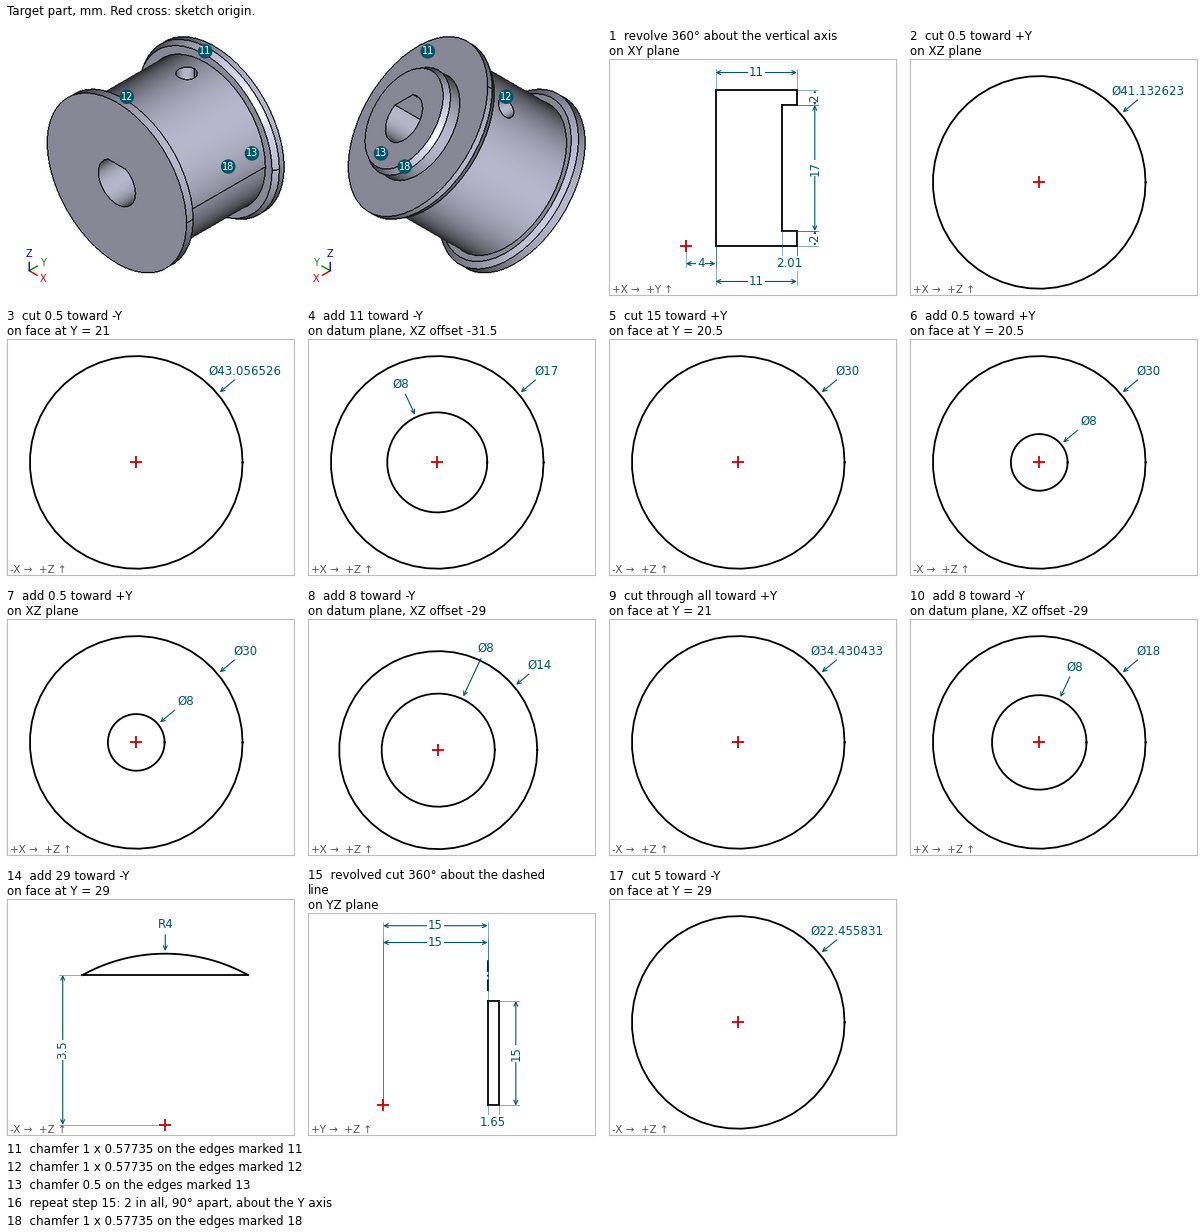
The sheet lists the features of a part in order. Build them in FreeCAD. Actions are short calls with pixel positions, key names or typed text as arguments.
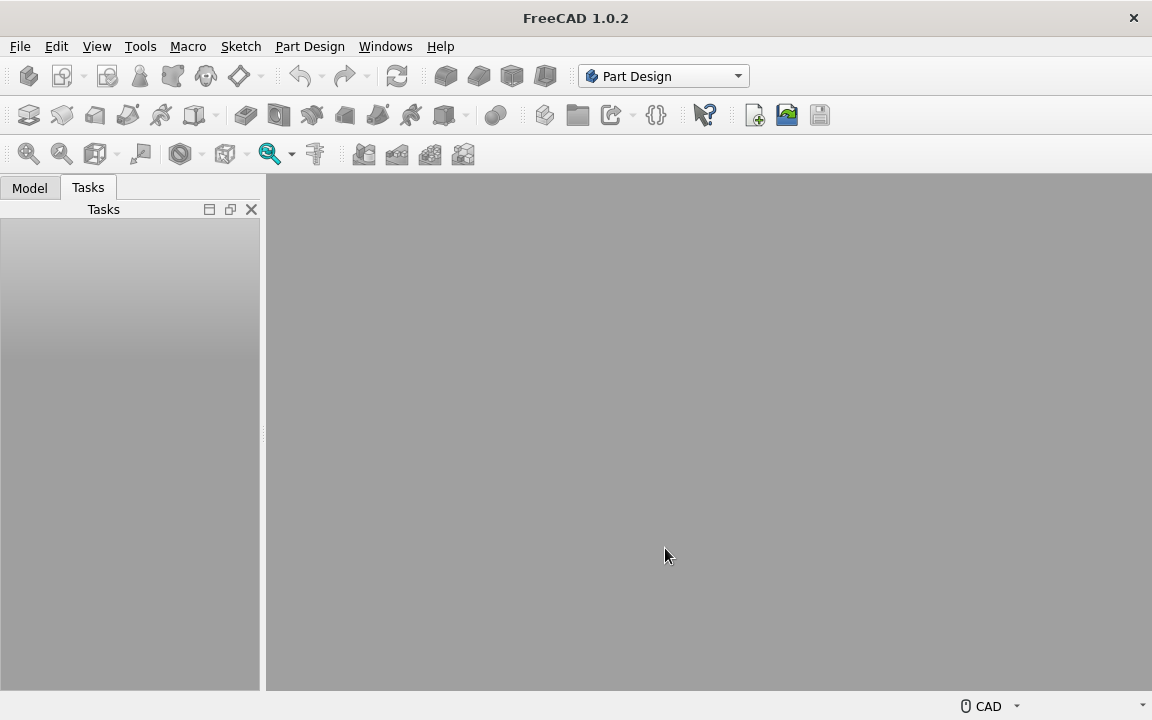
click(754, 116)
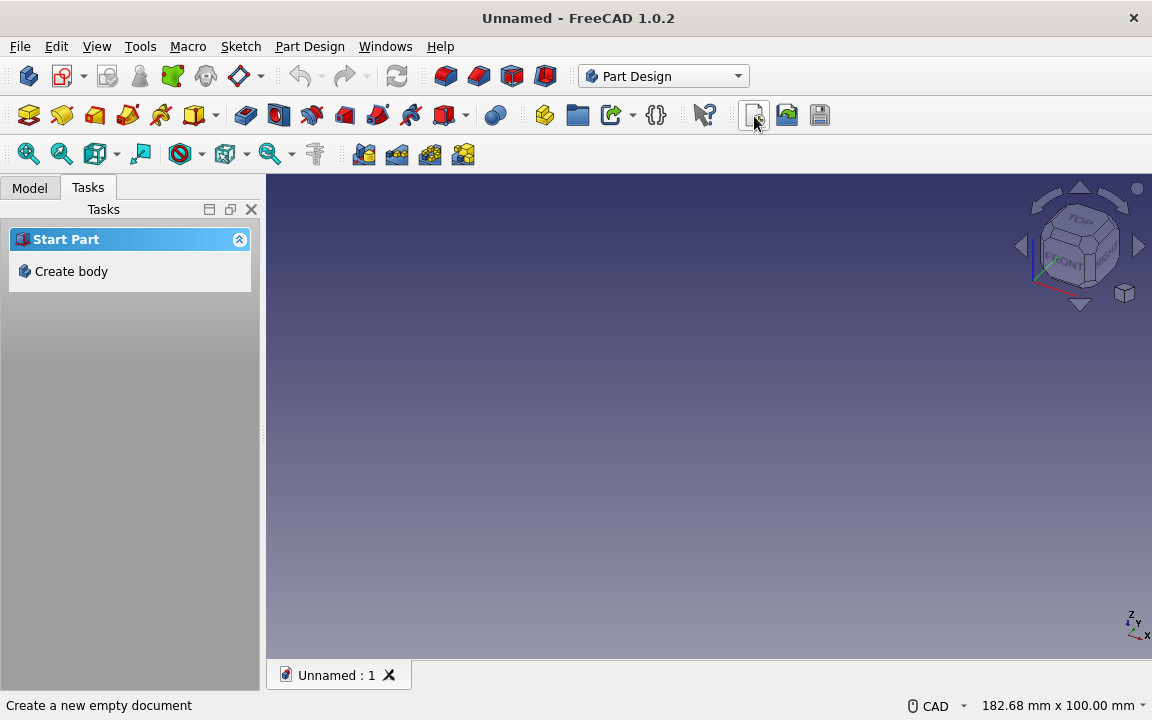
click(62, 76)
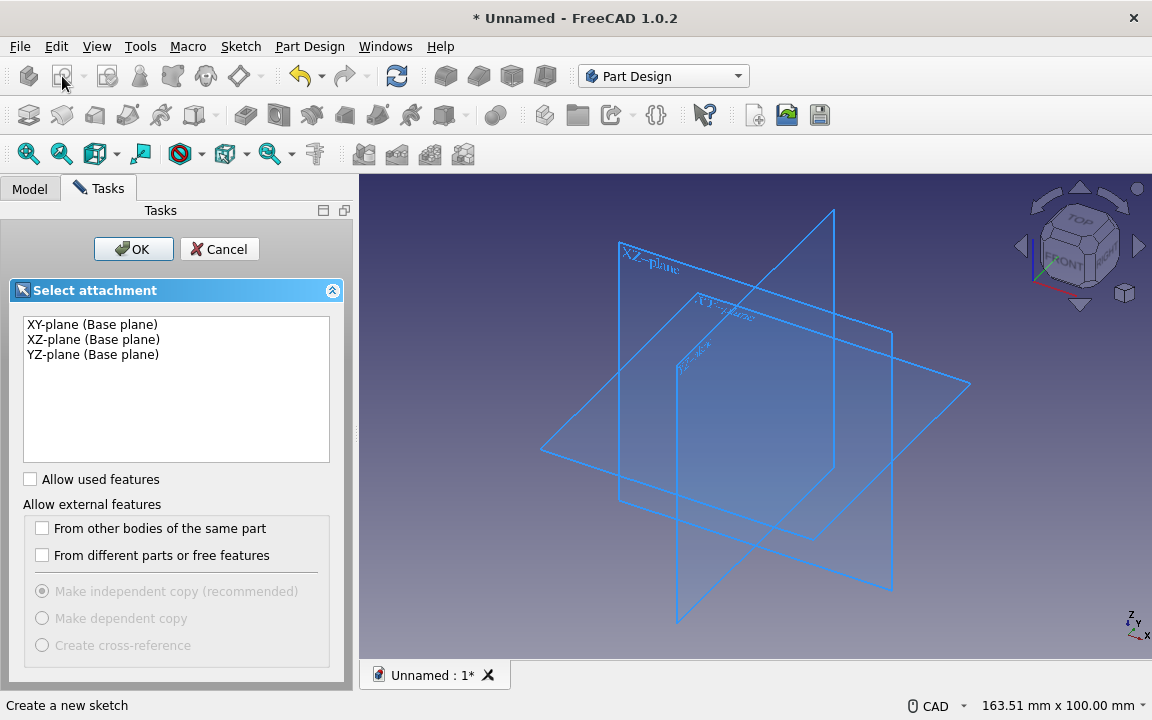
click(84, 324)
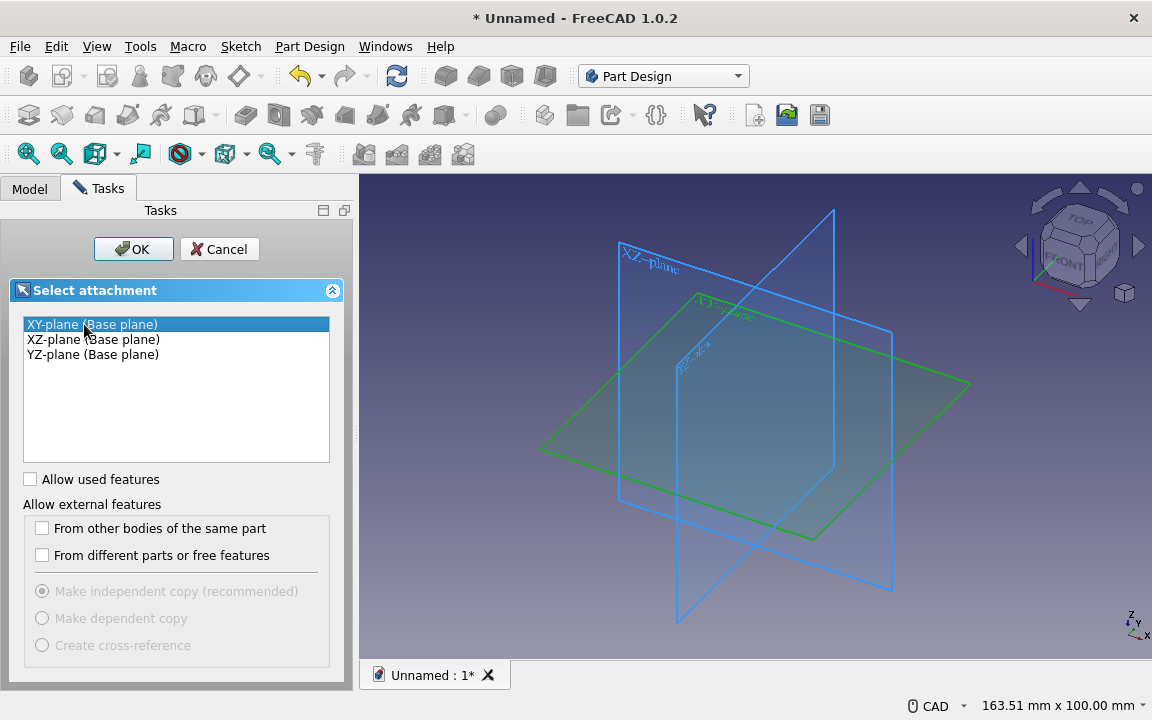
click(134, 249)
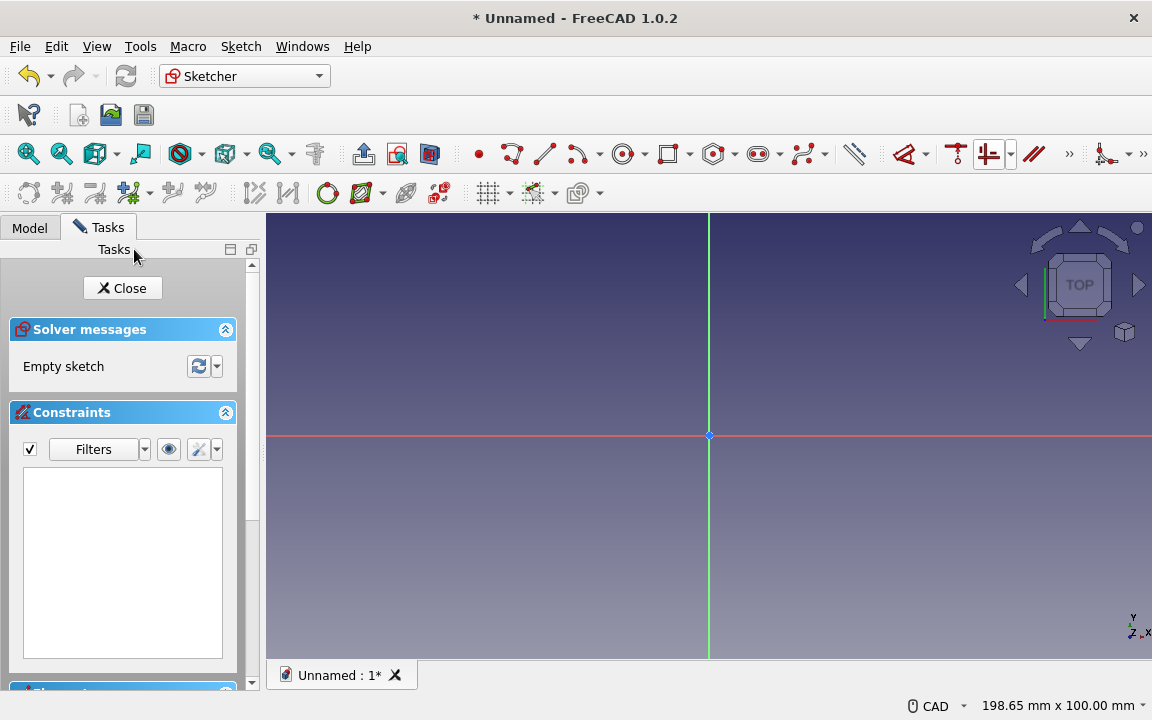
scroll(802, 362, up, 5)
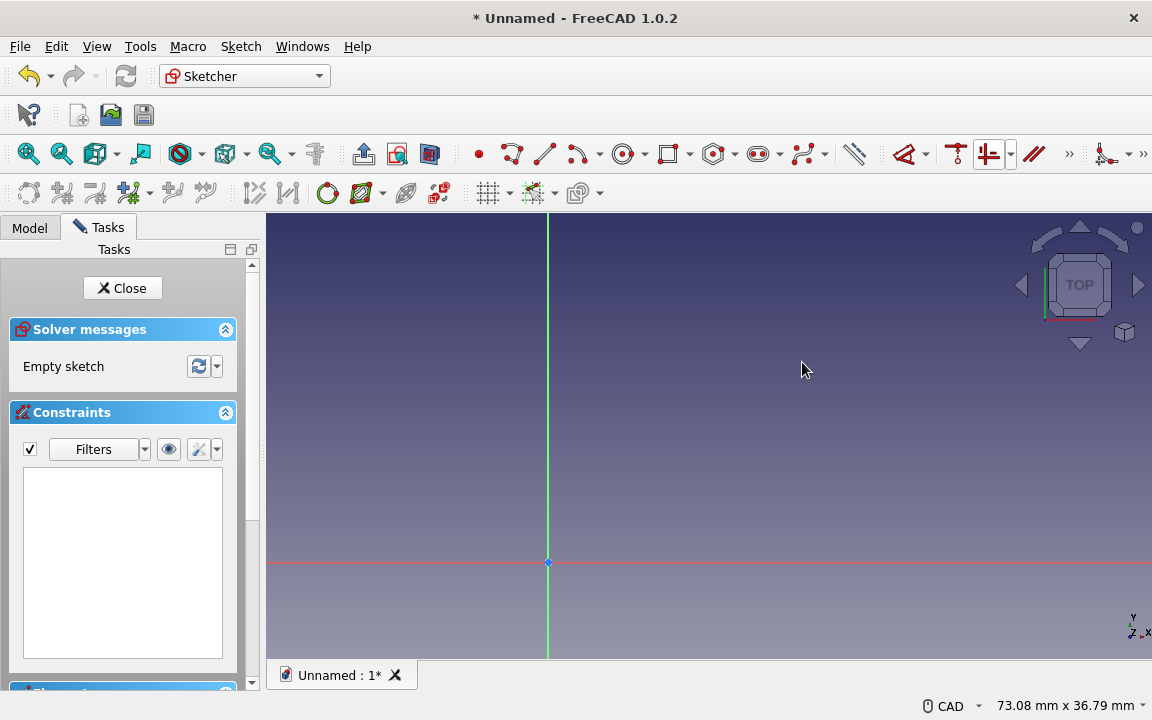
click(512, 154)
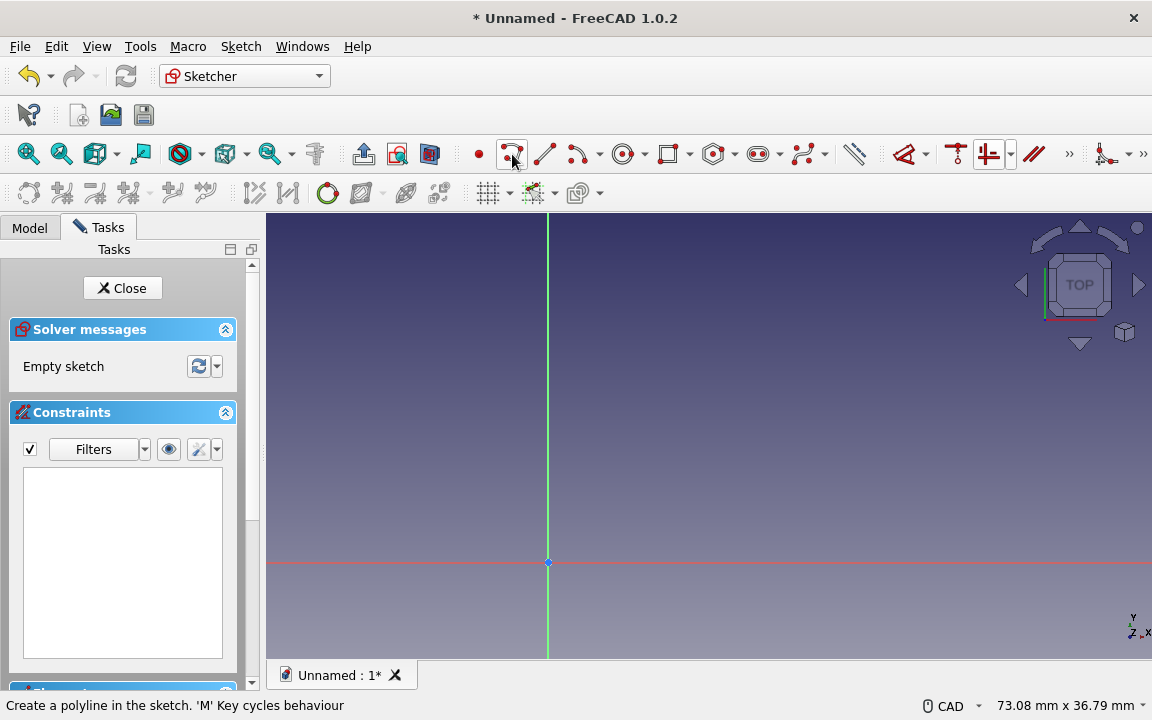
click(597, 563)
click(730, 554)
click(730, 538)
click(706, 538)
click(706, 332)
click(730, 332)
click(730, 308)
click(597, 308)
click(597, 563)
key(Escape)
key(Escape)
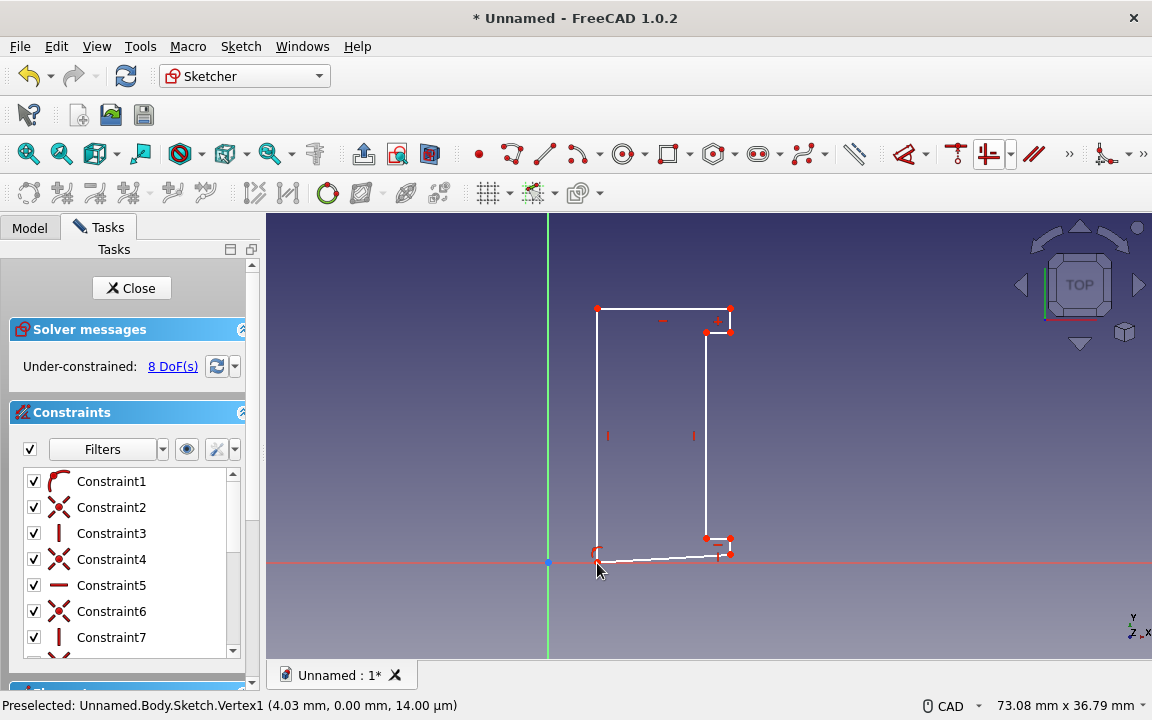
click(637, 560)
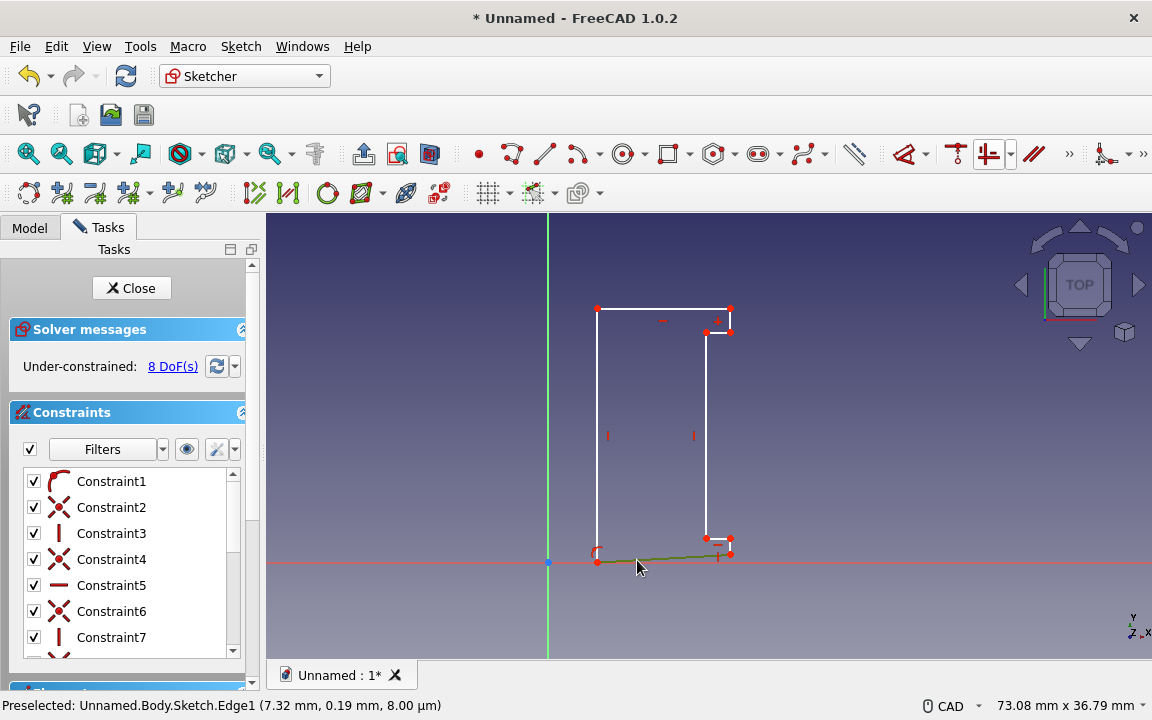
click(1010, 154)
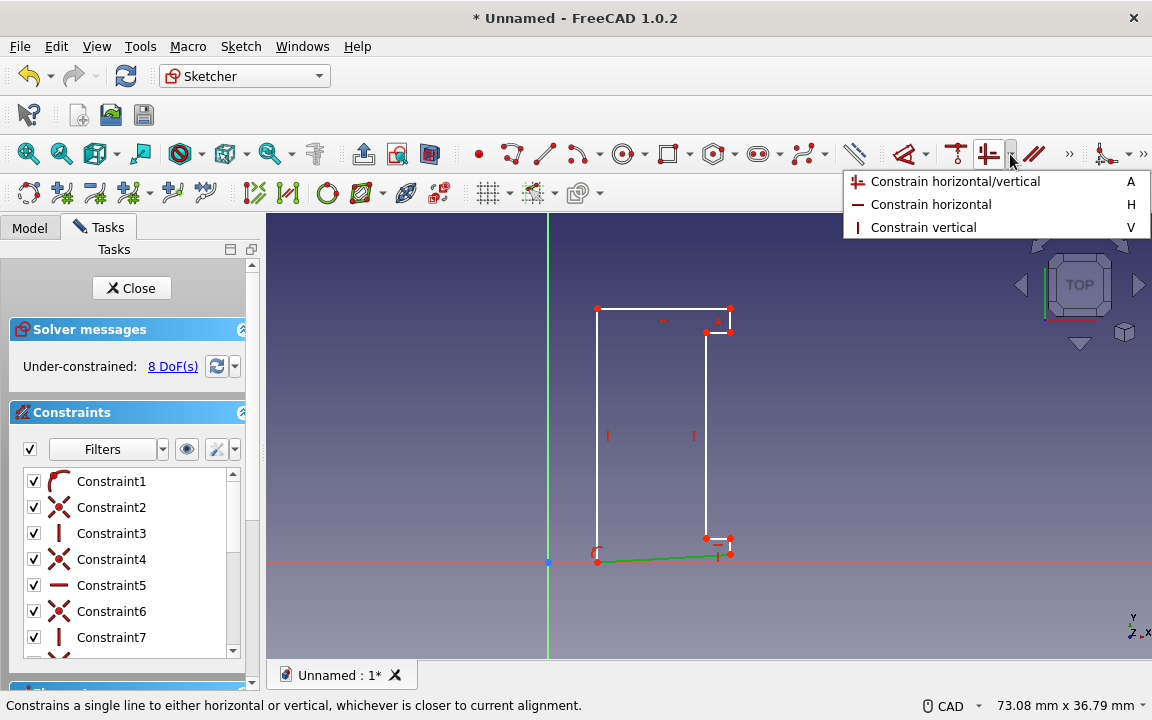
click(997, 204)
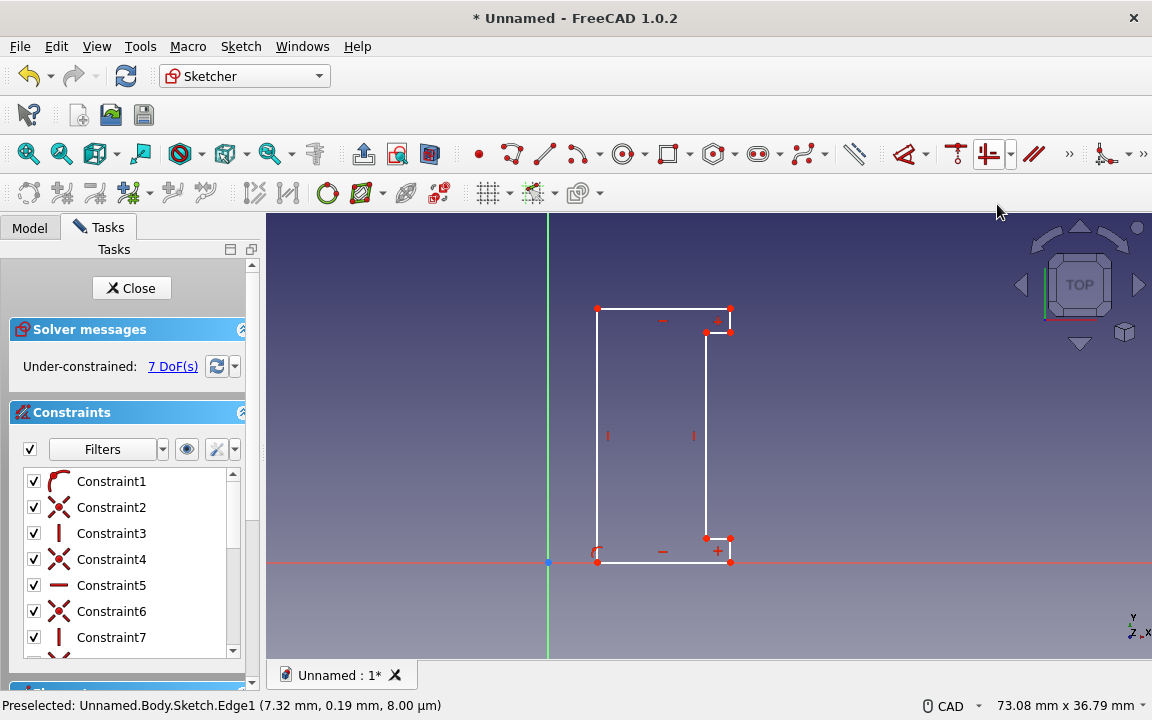
click(904, 154)